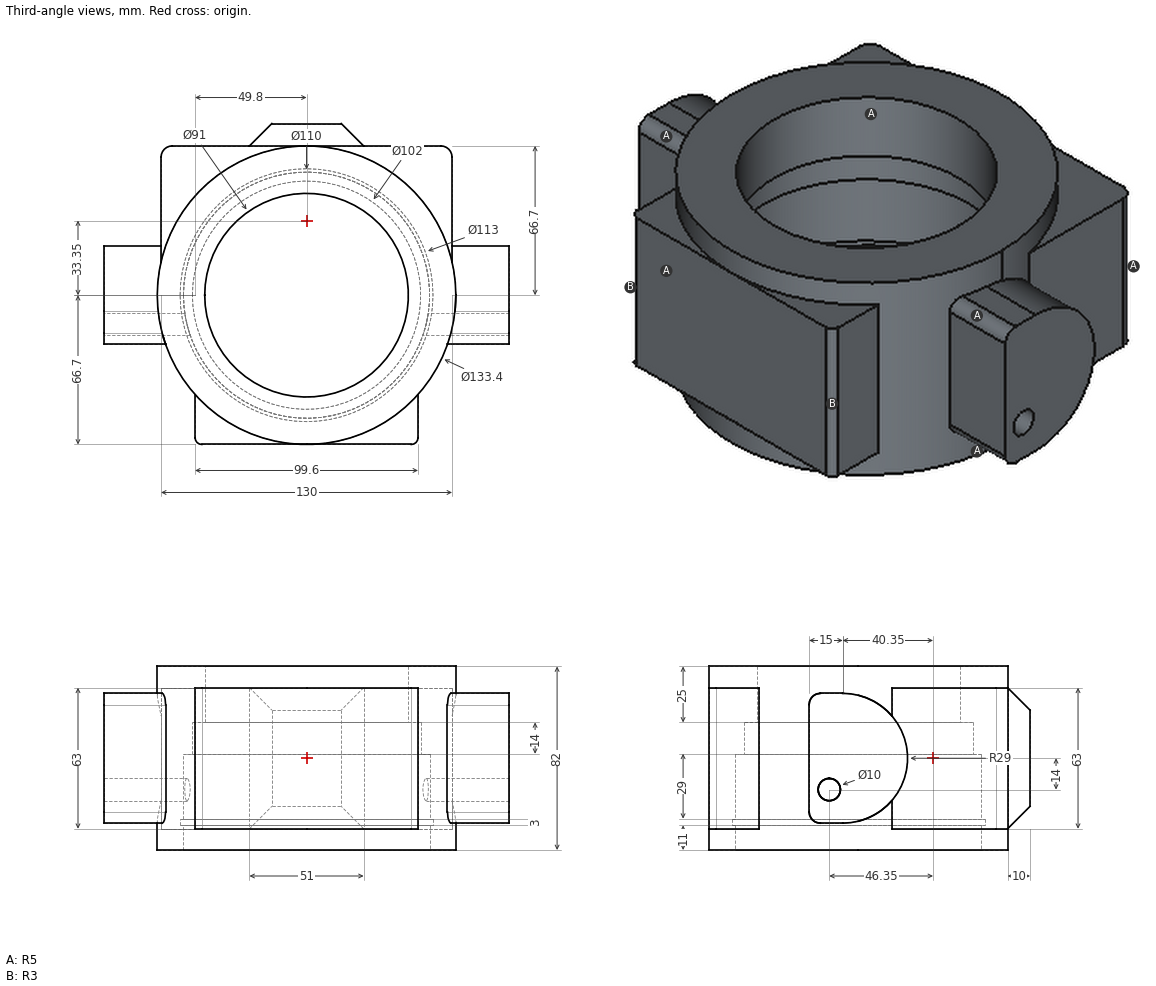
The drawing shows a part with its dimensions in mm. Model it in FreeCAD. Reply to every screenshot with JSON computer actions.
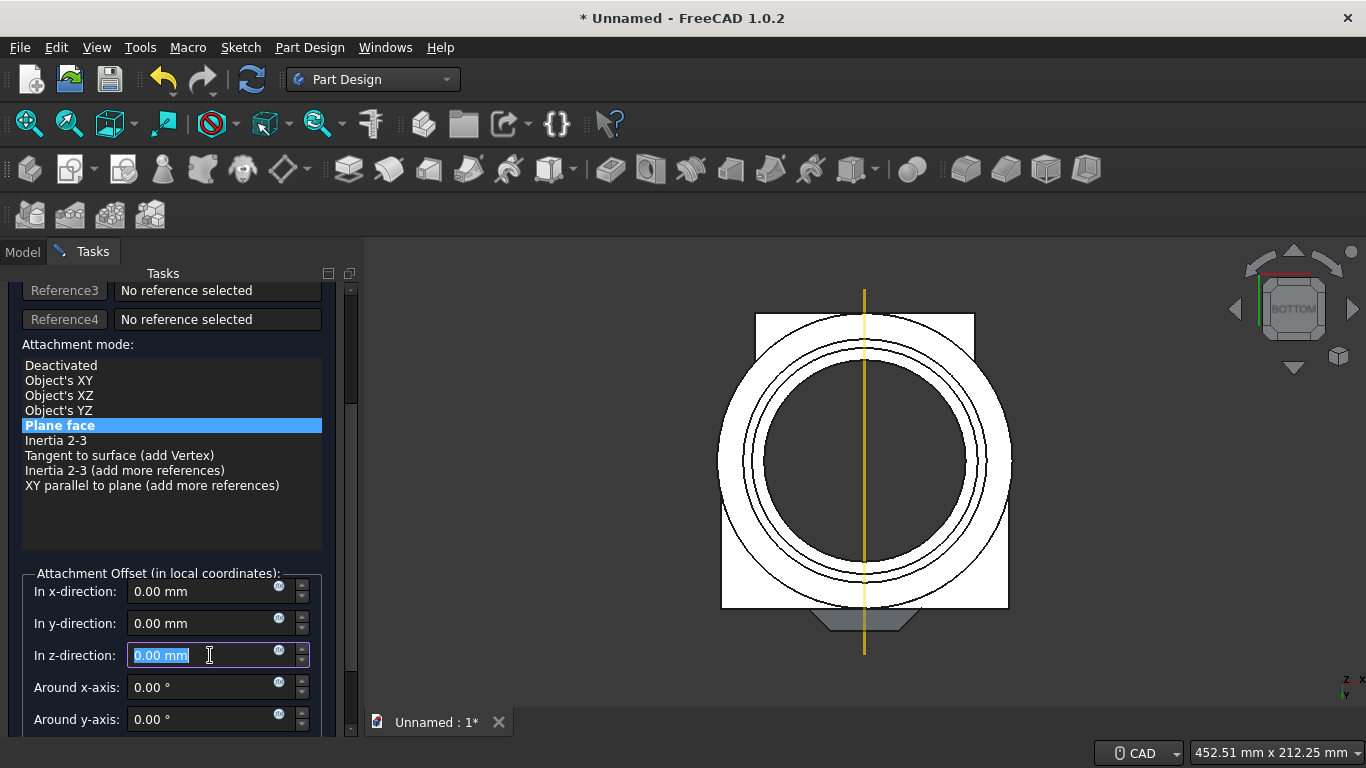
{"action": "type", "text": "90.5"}
{"action": "key", "text": "Tab"}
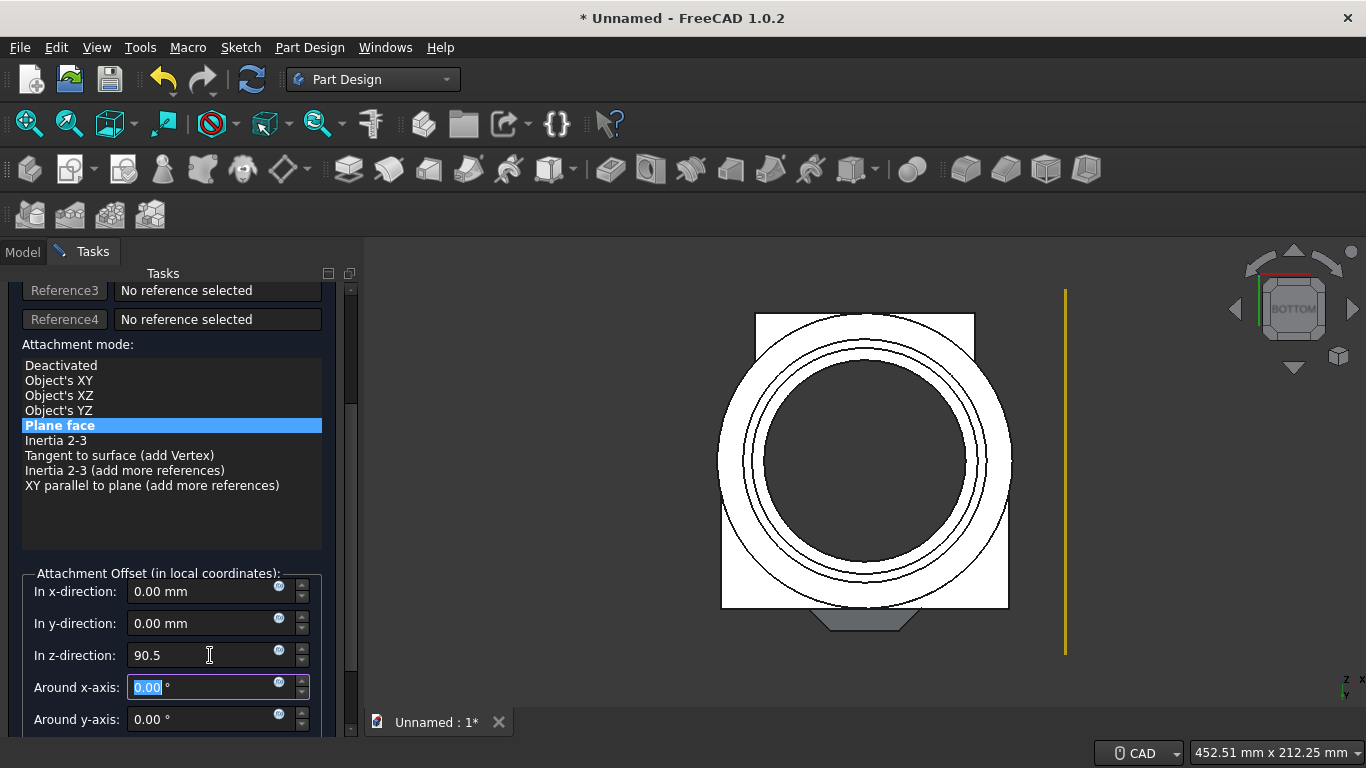
{"action": "scroll", "coordinate": [351, 510], "scroll_direction": "up", "scroll_amount": 4}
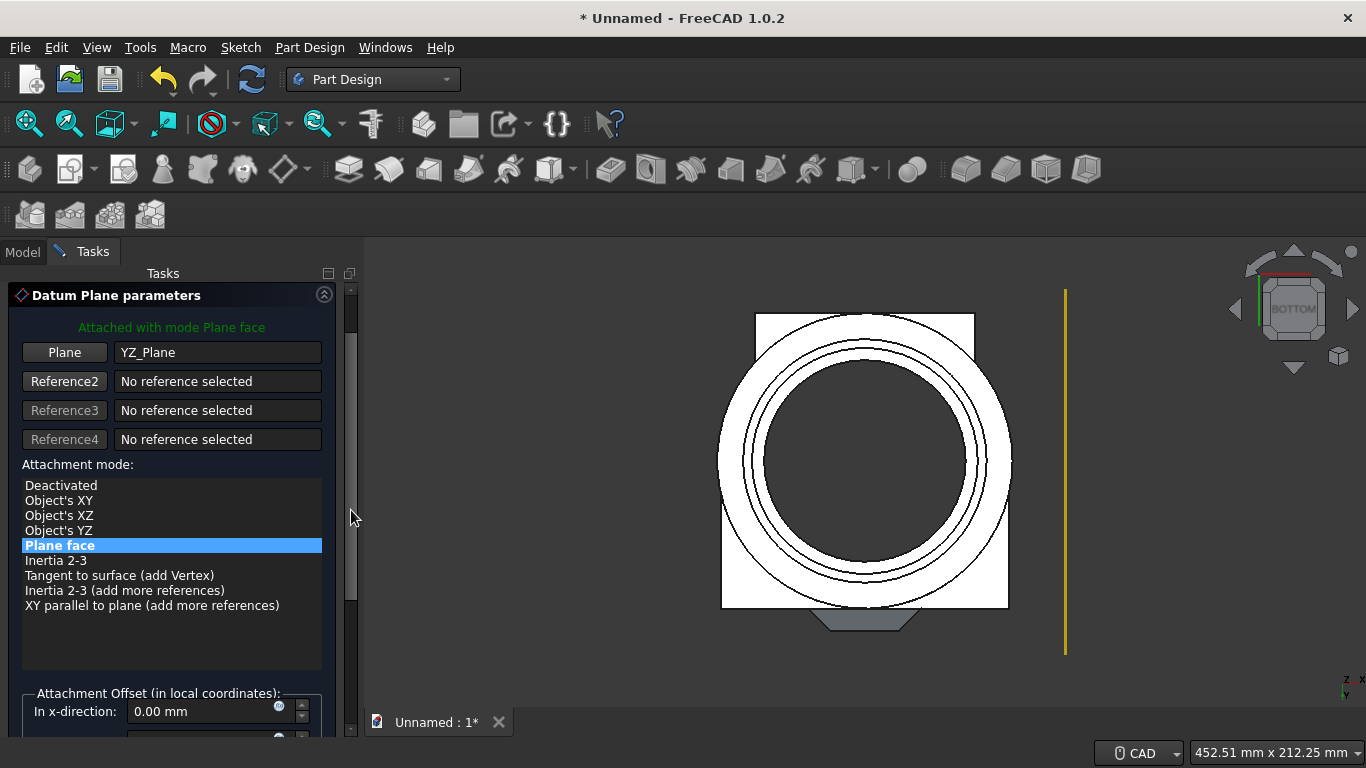
{"action": "left_click", "coordinate": [124, 312]}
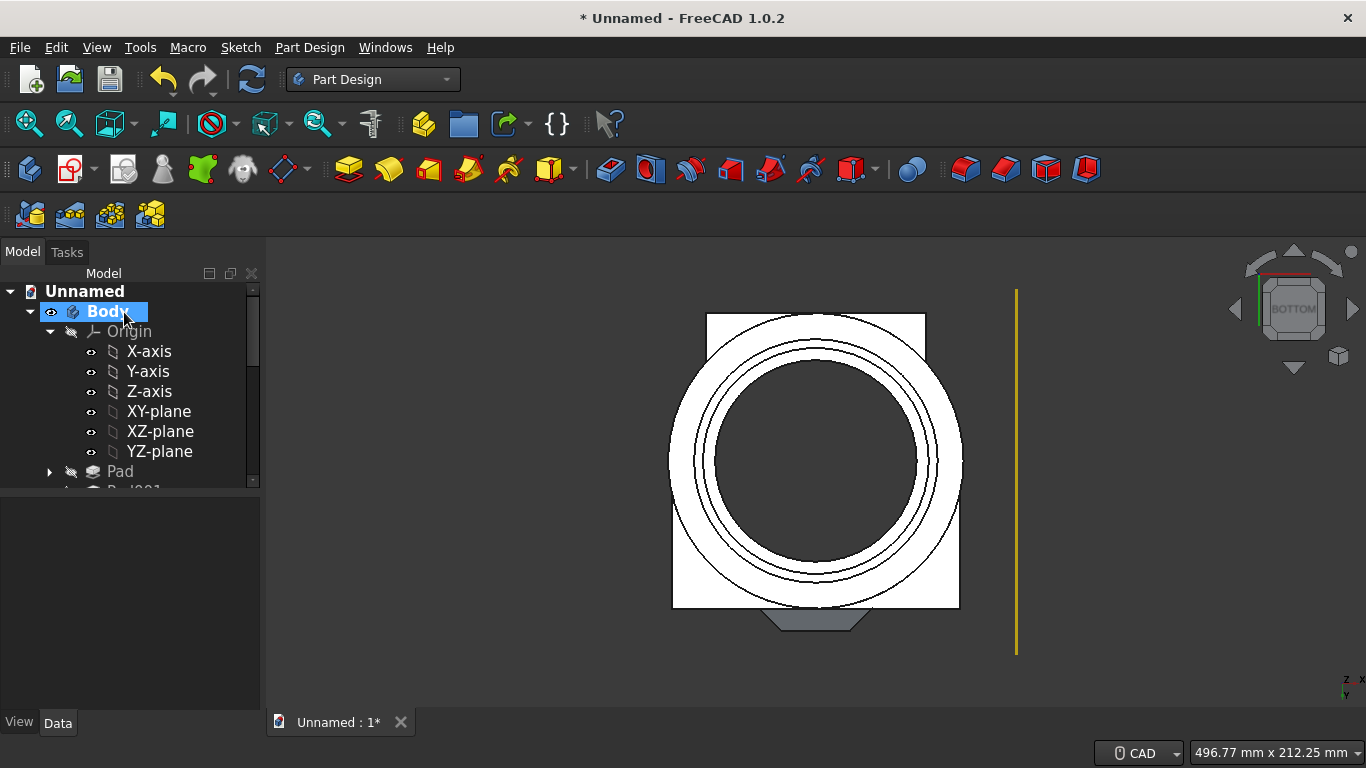
{"action": "scroll", "coordinate": [100, 387], "scroll_direction": "down", "scroll_amount": 3}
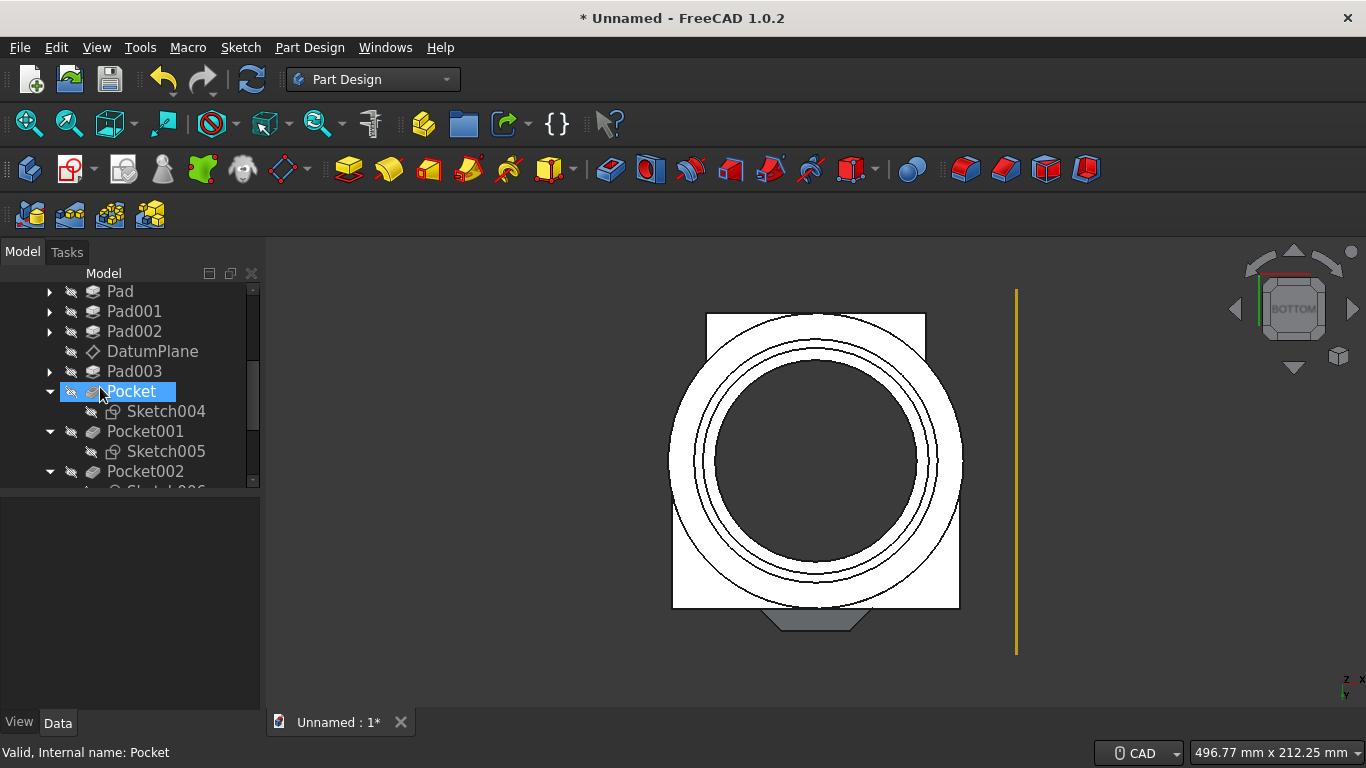
{"action": "scroll", "coordinate": [140, 387], "scroll_direction": "up", "scroll_amount": 15}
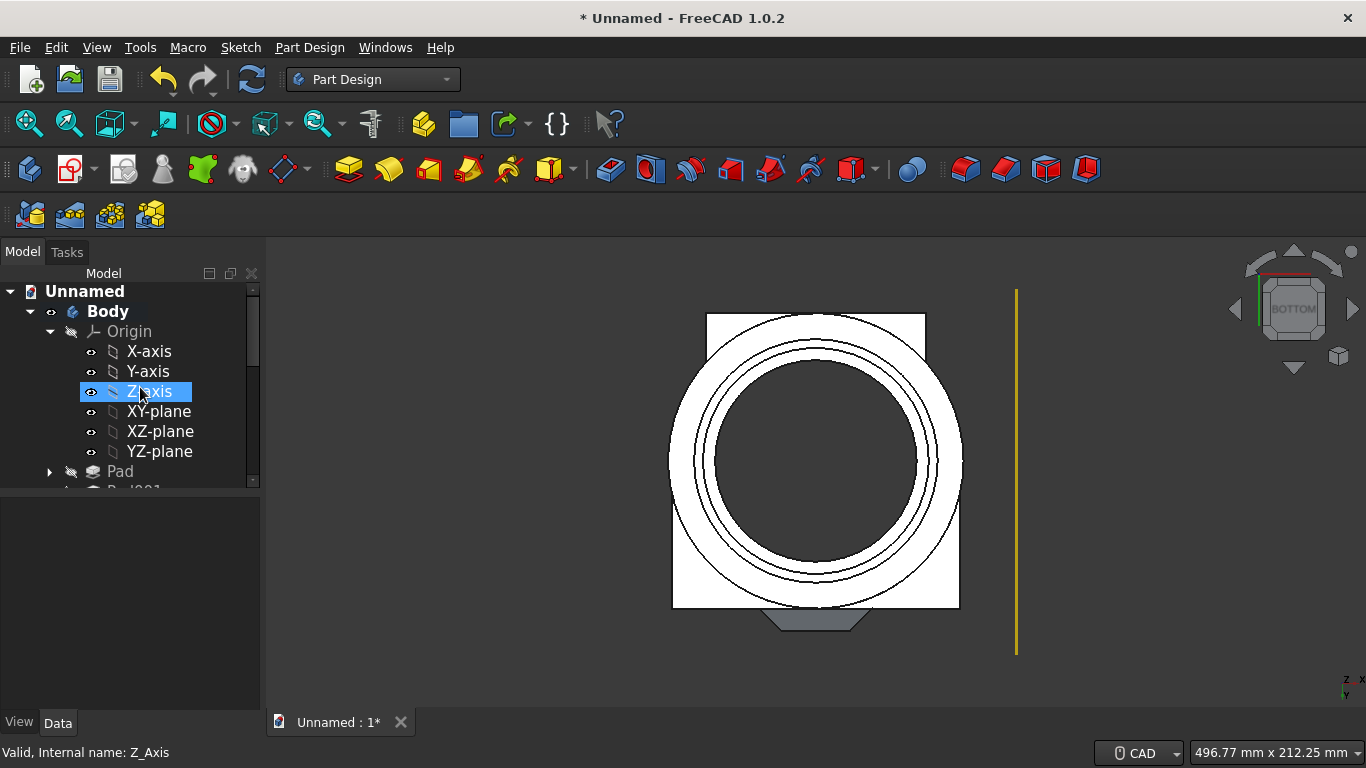
{"action": "scroll", "coordinate": [100, 387], "scroll_direction": "down", "scroll_amount": 6}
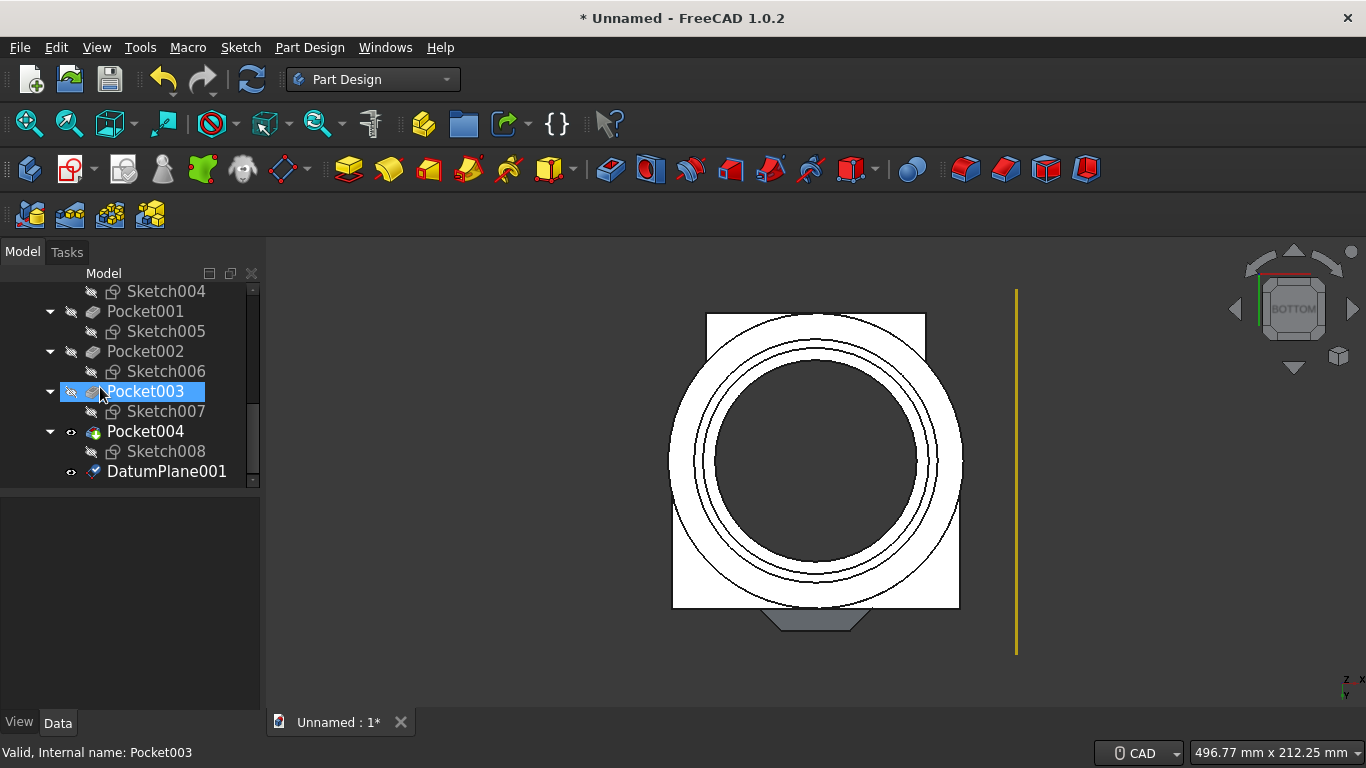
{"action": "left_click", "coordinate": [116, 472]}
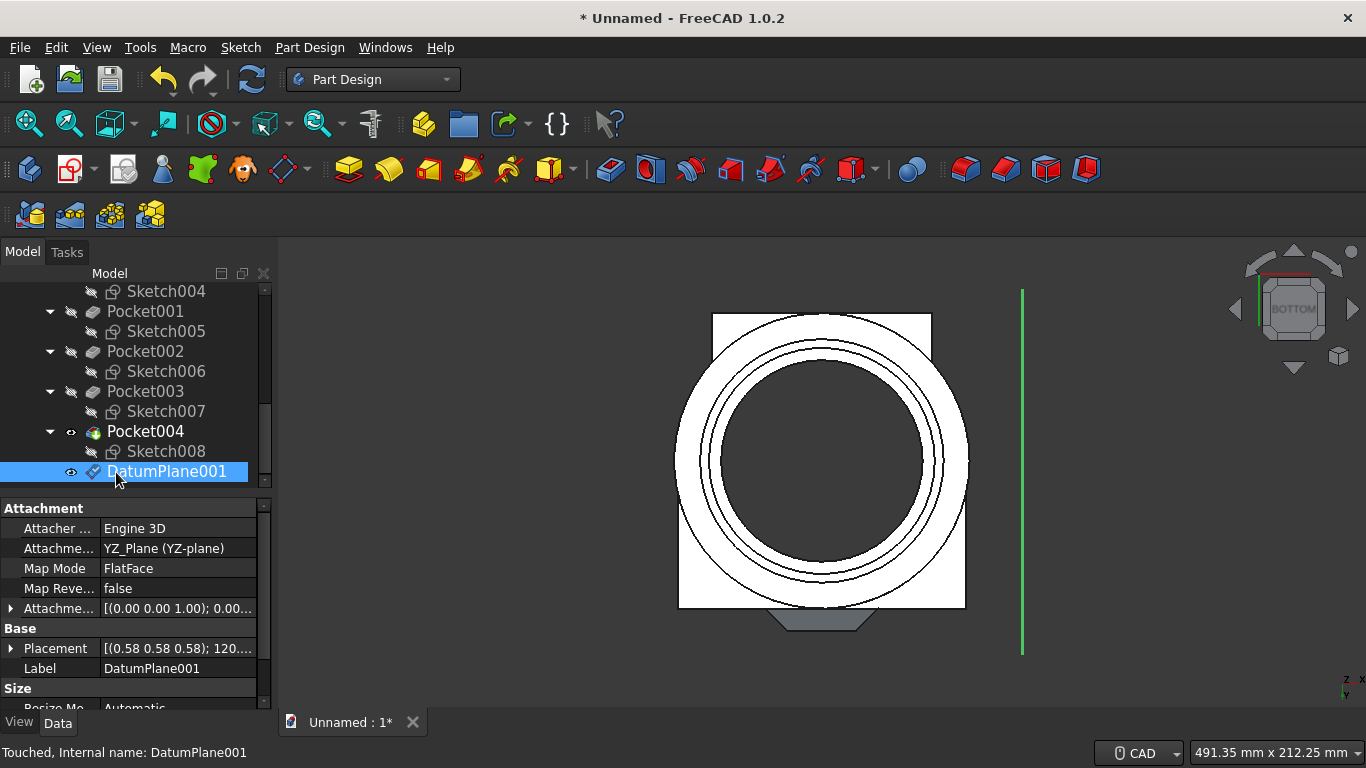
{"action": "left_click", "coordinate": [70, 170]}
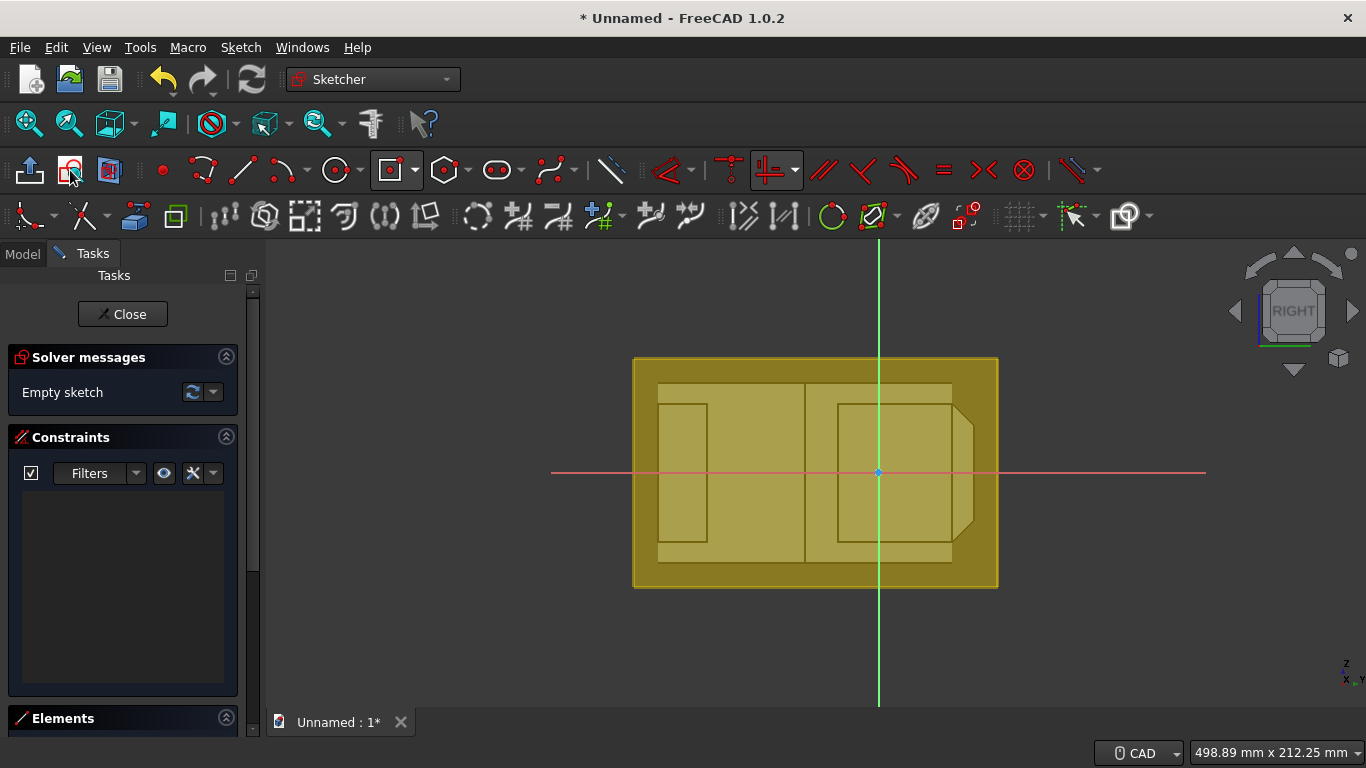
{"action": "scroll", "coordinate": [875, 473], "scroll_direction": "up", "scroll_amount": 4}